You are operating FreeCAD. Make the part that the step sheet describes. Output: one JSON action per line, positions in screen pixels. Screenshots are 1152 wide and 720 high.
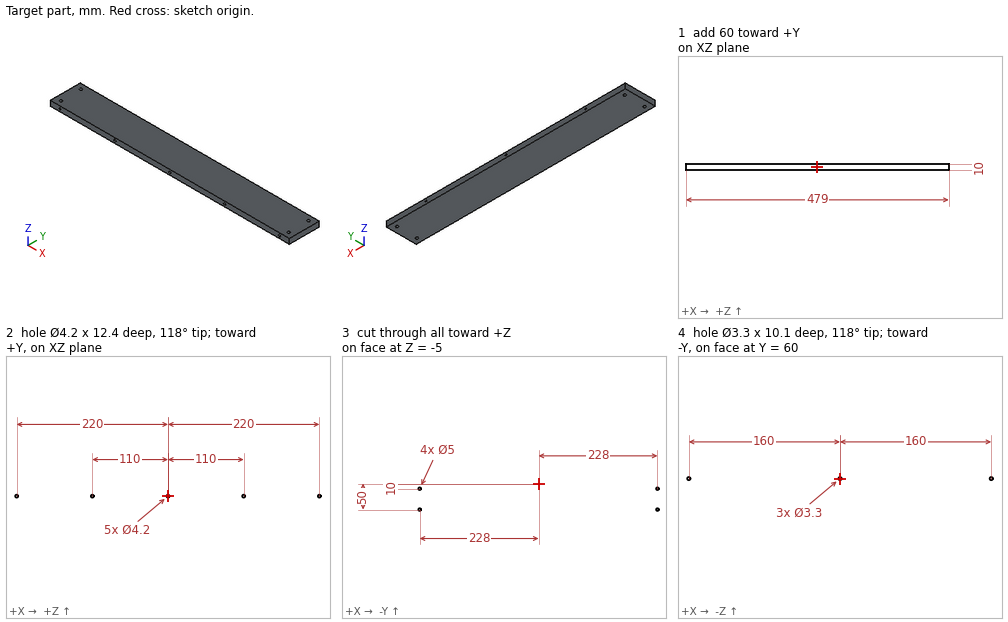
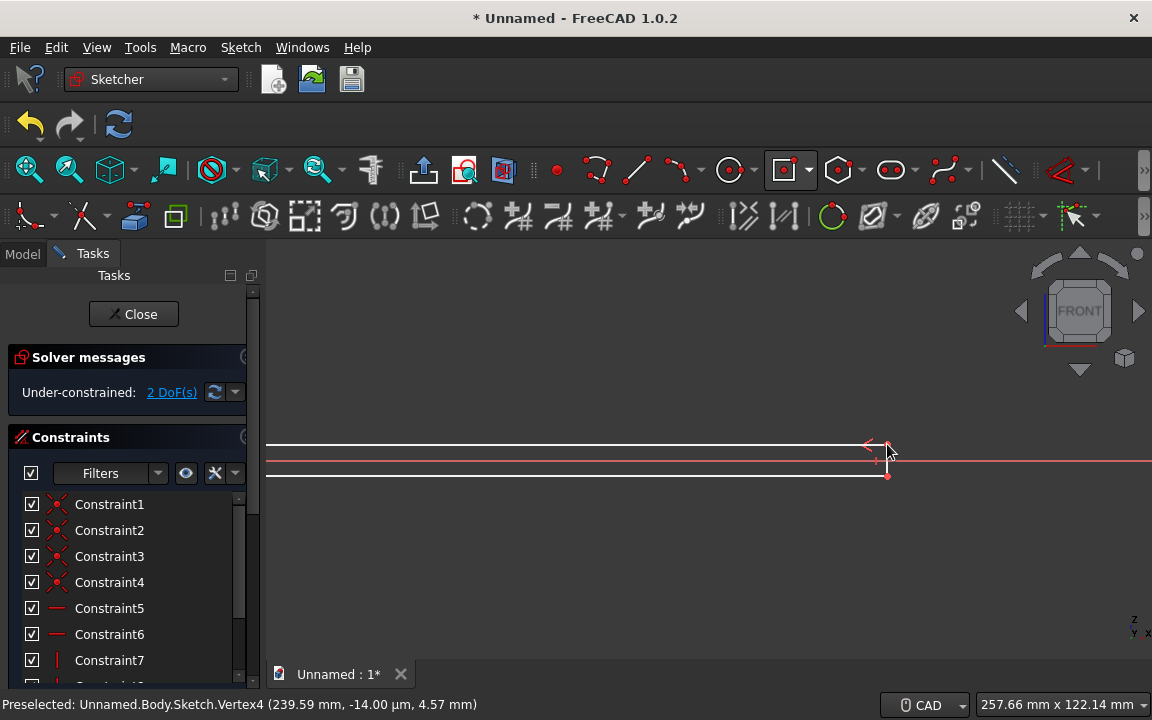
{"action": "left_click", "coordinate": [1060, 170]}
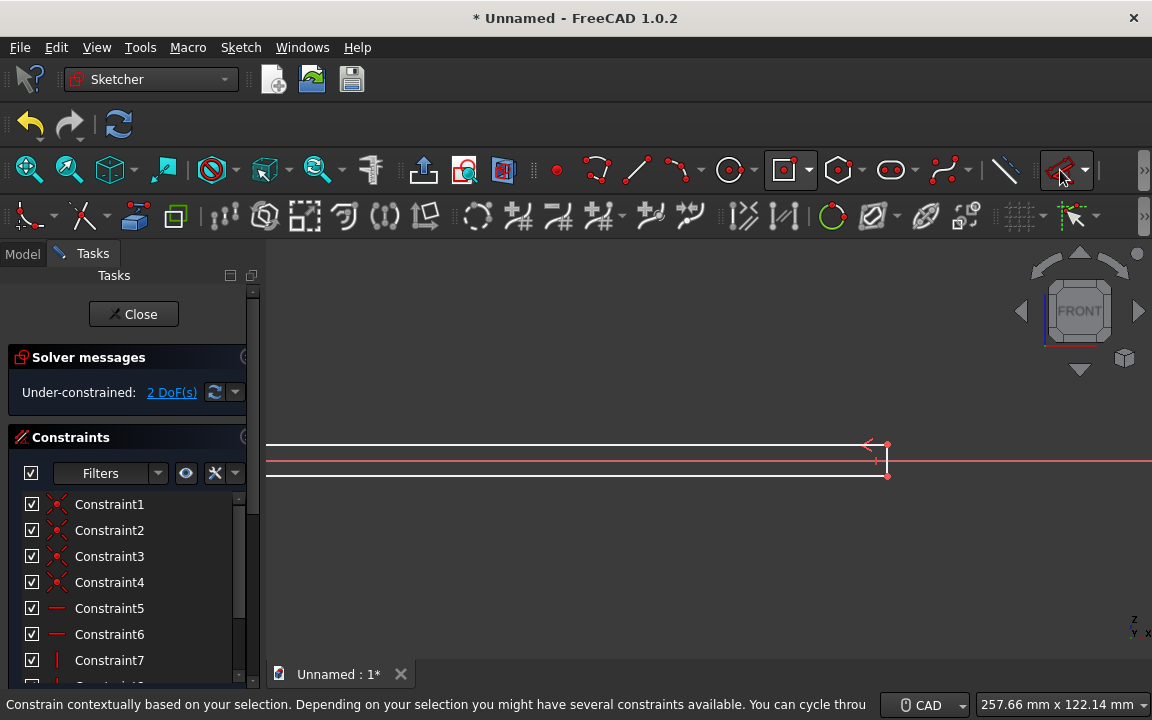
{"action": "left_click", "coordinate": [887, 464]}
{"action": "left_click", "coordinate": [921, 453]}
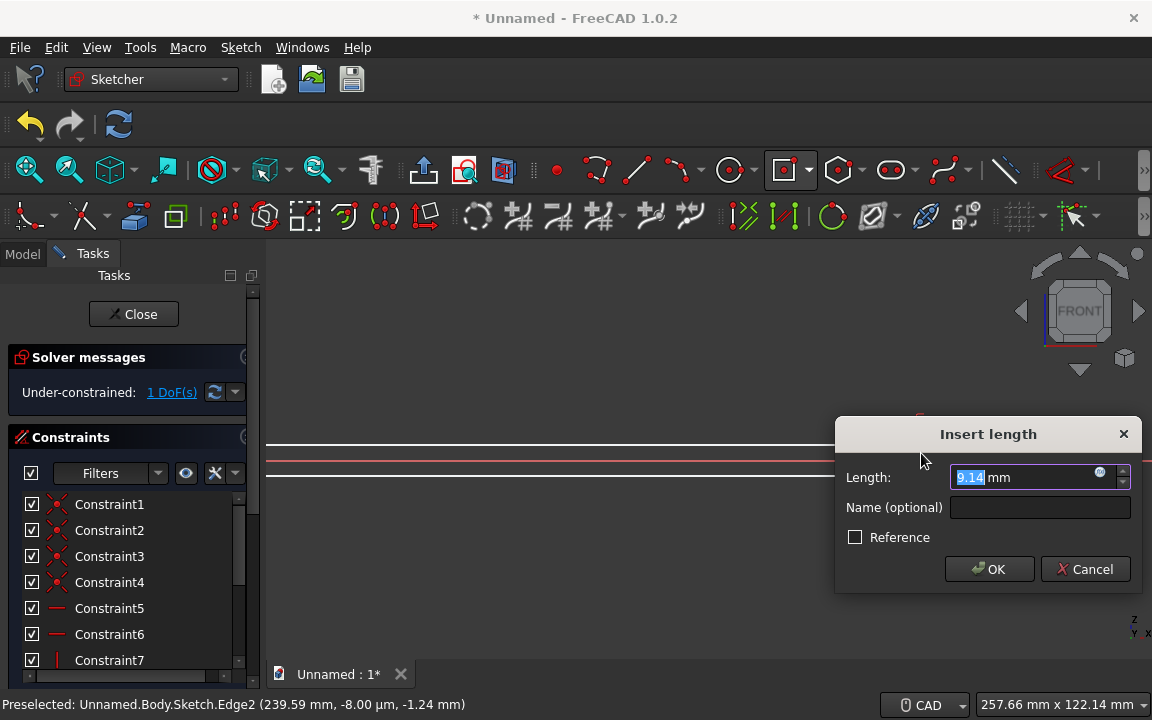
{"action": "type", "text": "10"}
{"action": "key", "text": "Return"}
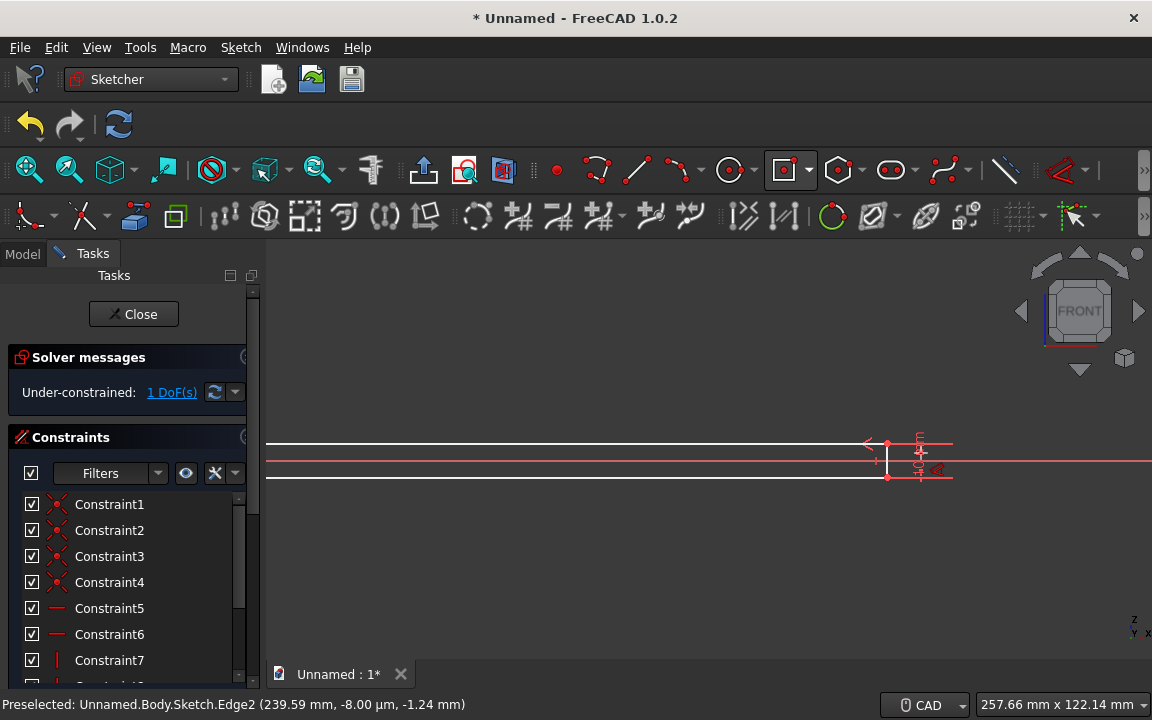
{"action": "left_click", "coordinate": [393, 478]}
{"action": "left_click", "coordinate": [590, 512]}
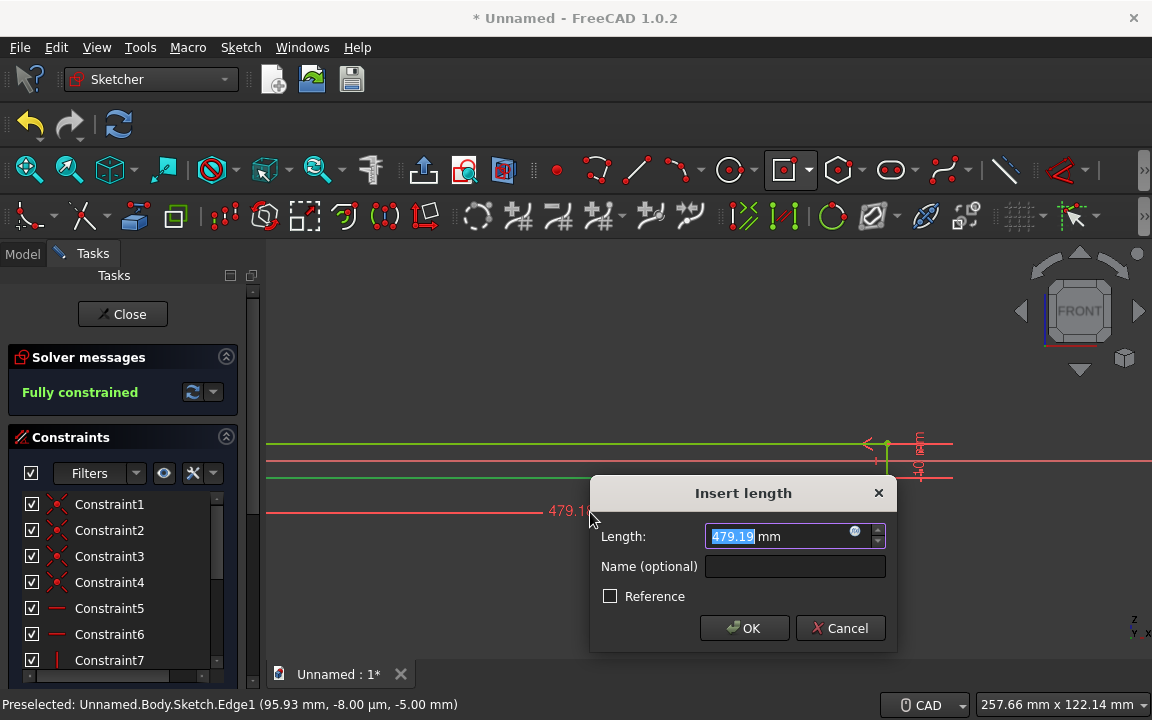
{"action": "type", "text": "479"}
{"action": "key", "text": "Return"}
{"action": "key", "text": "Escape"}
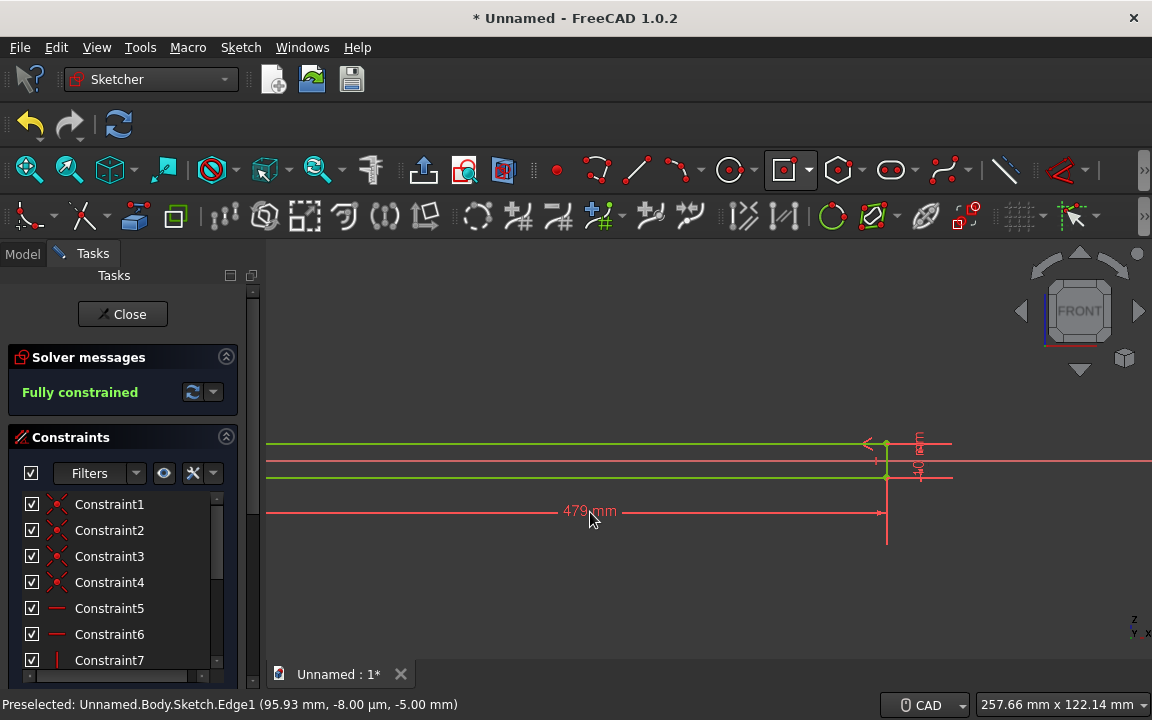
{"action": "left_click", "coordinate": [123, 314]}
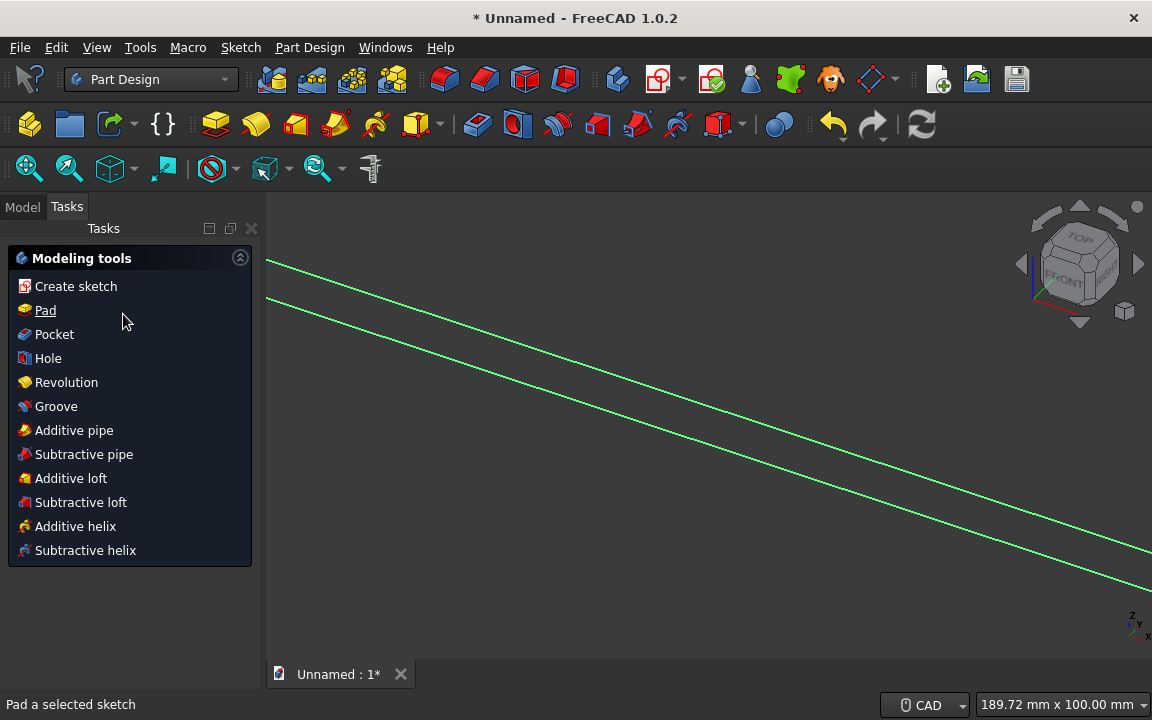
{"action": "left_click", "coordinate": [216, 124]}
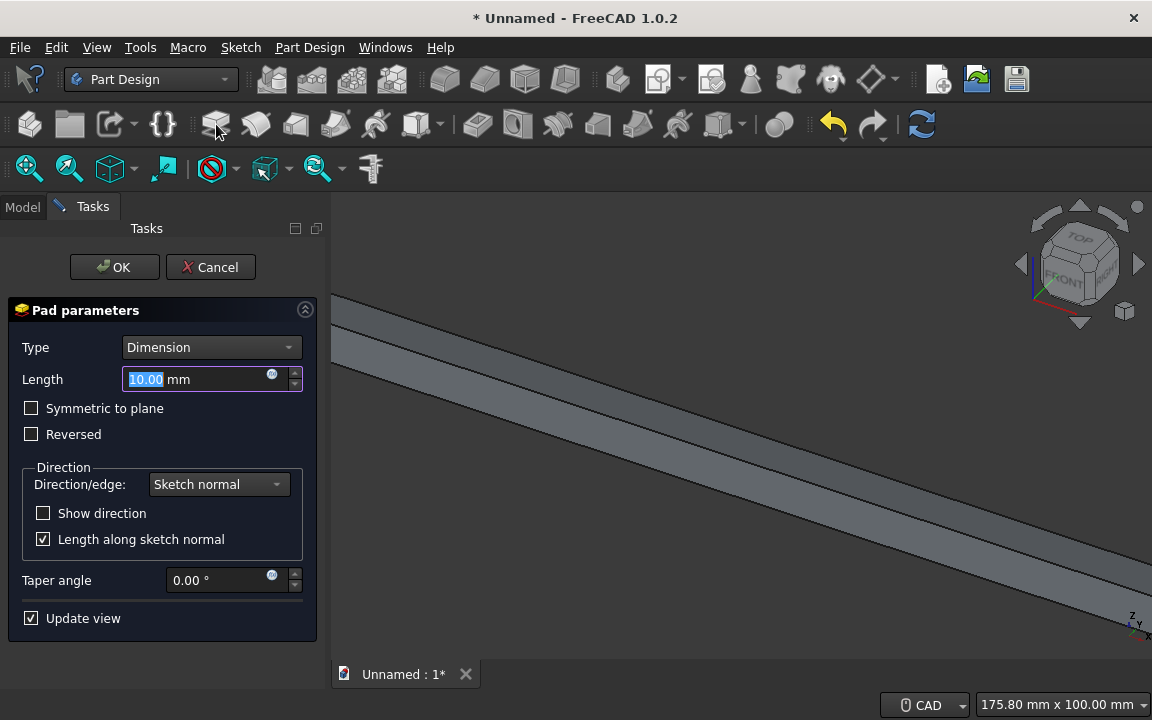
{"action": "type", "text": "60"}
{"action": "key", "text": "Tab"}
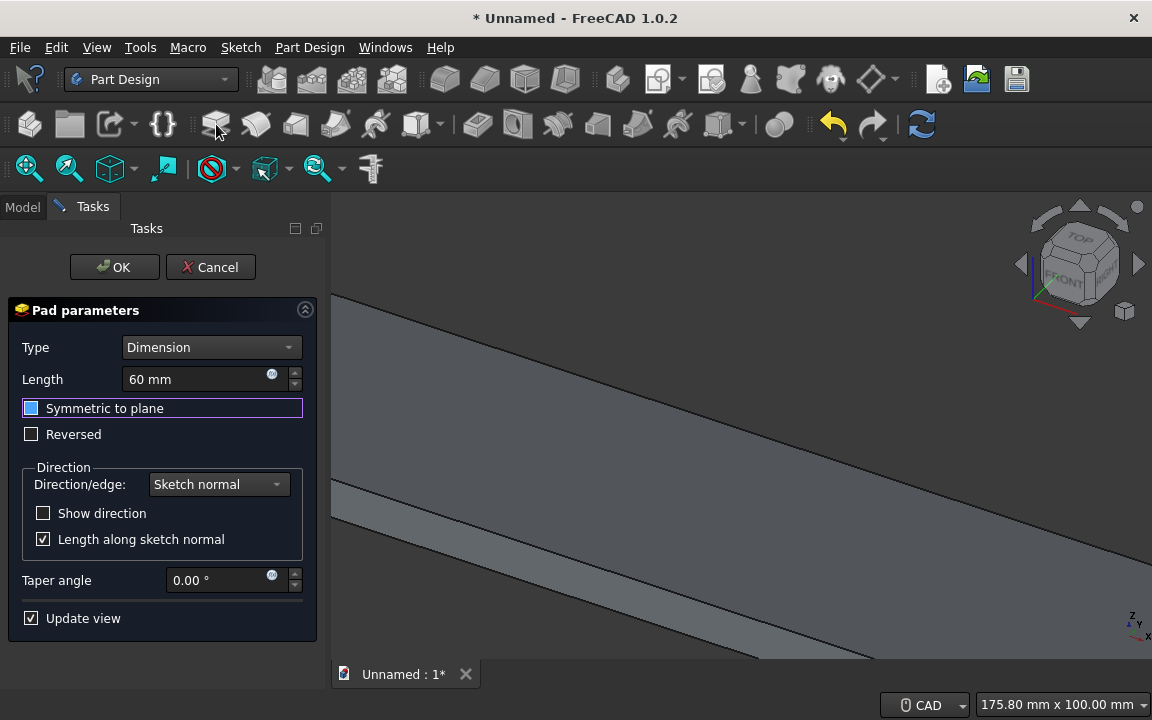
{"action": "left_click", "coordinate": [30, 434]}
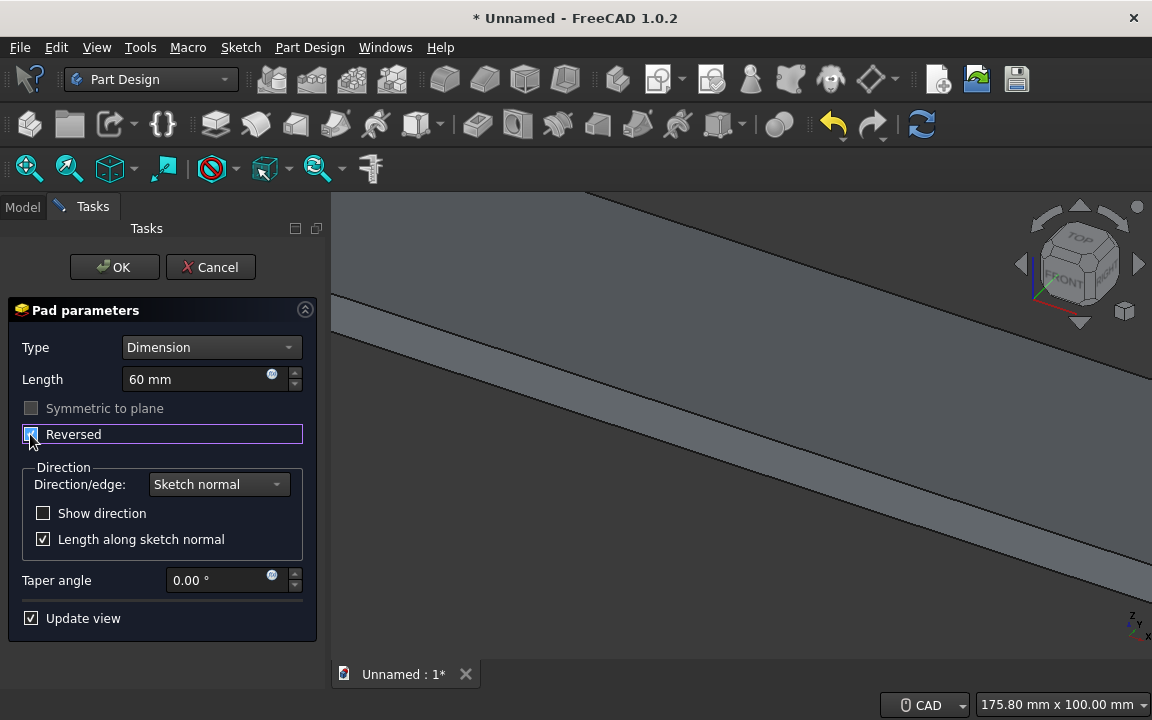
{"action": "left_click", "coordinate": [115, 267]}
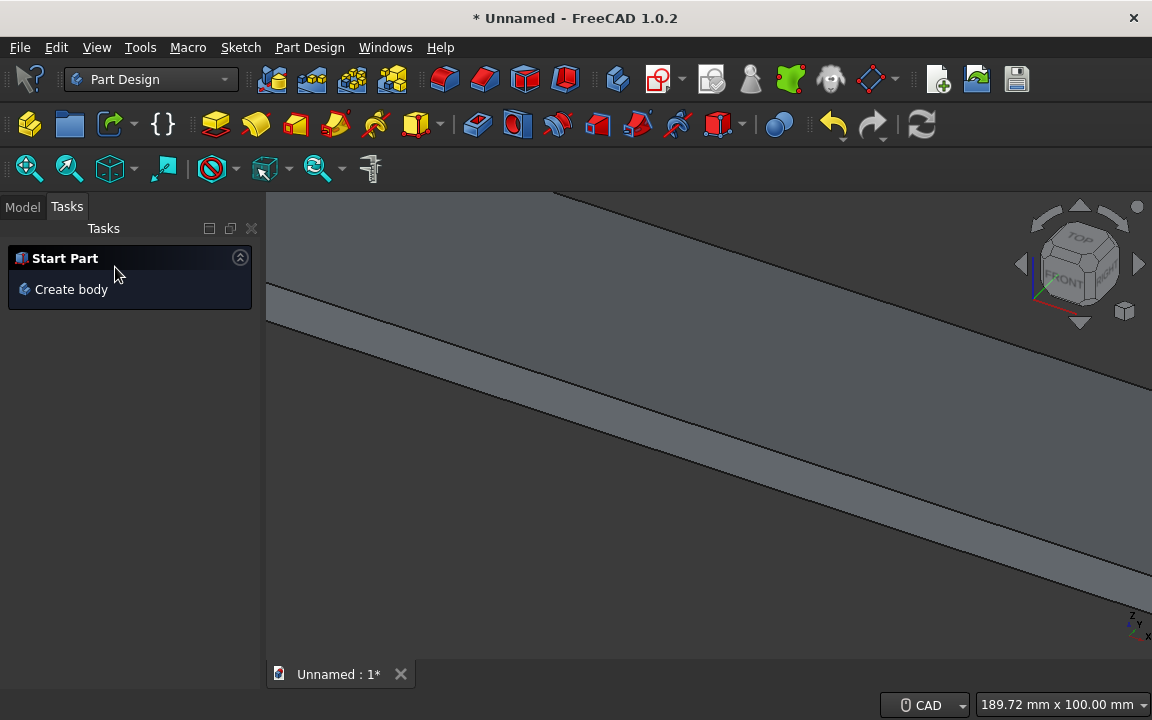
{"action": "key", "text": "v f"}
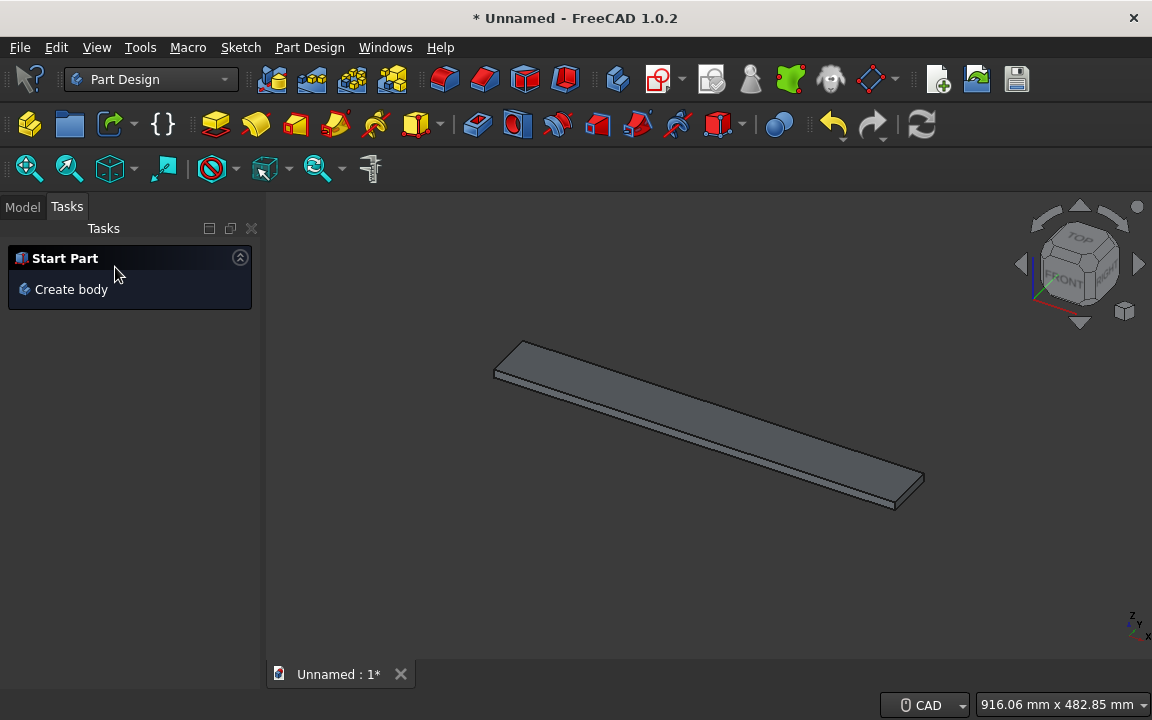
{"action": "left_click", "coordinate": [658, 80]}